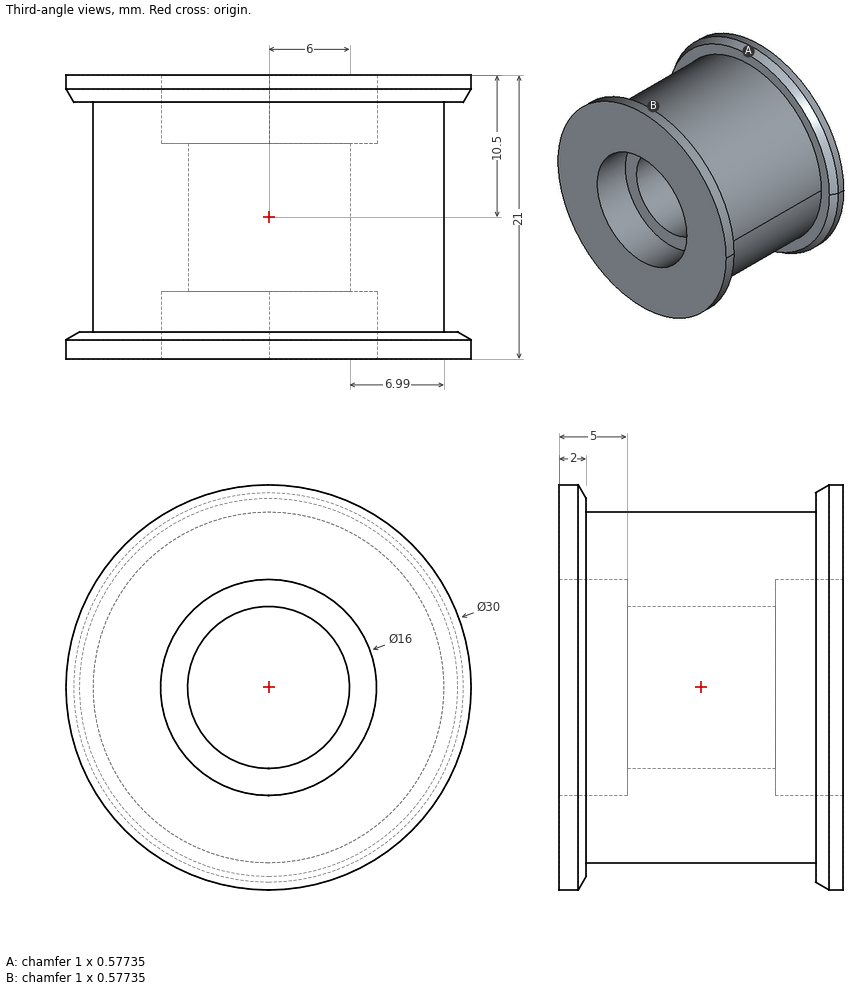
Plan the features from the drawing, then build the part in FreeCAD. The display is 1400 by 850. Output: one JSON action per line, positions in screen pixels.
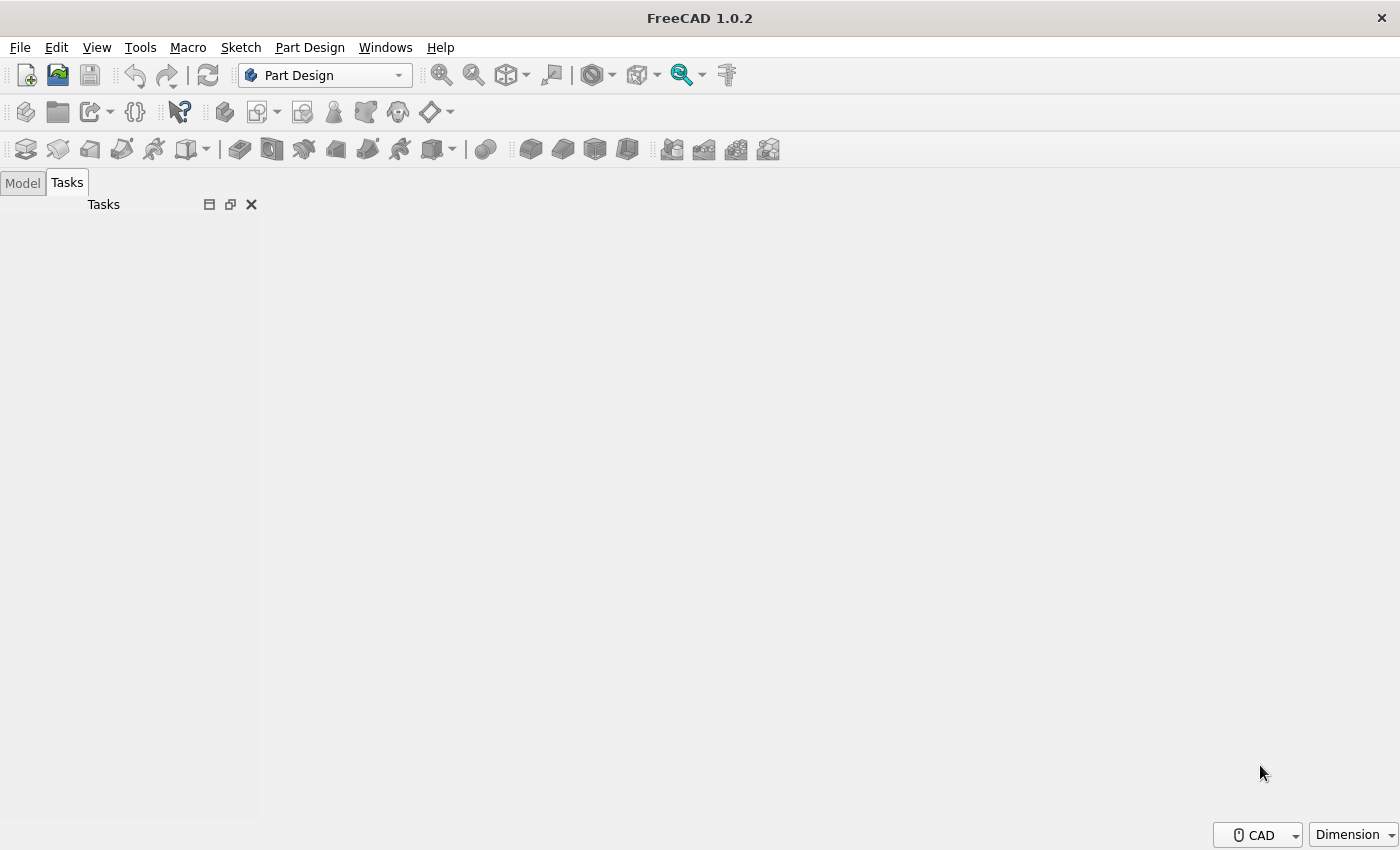
{"action": "left_click", "coordinate": [26, 76]}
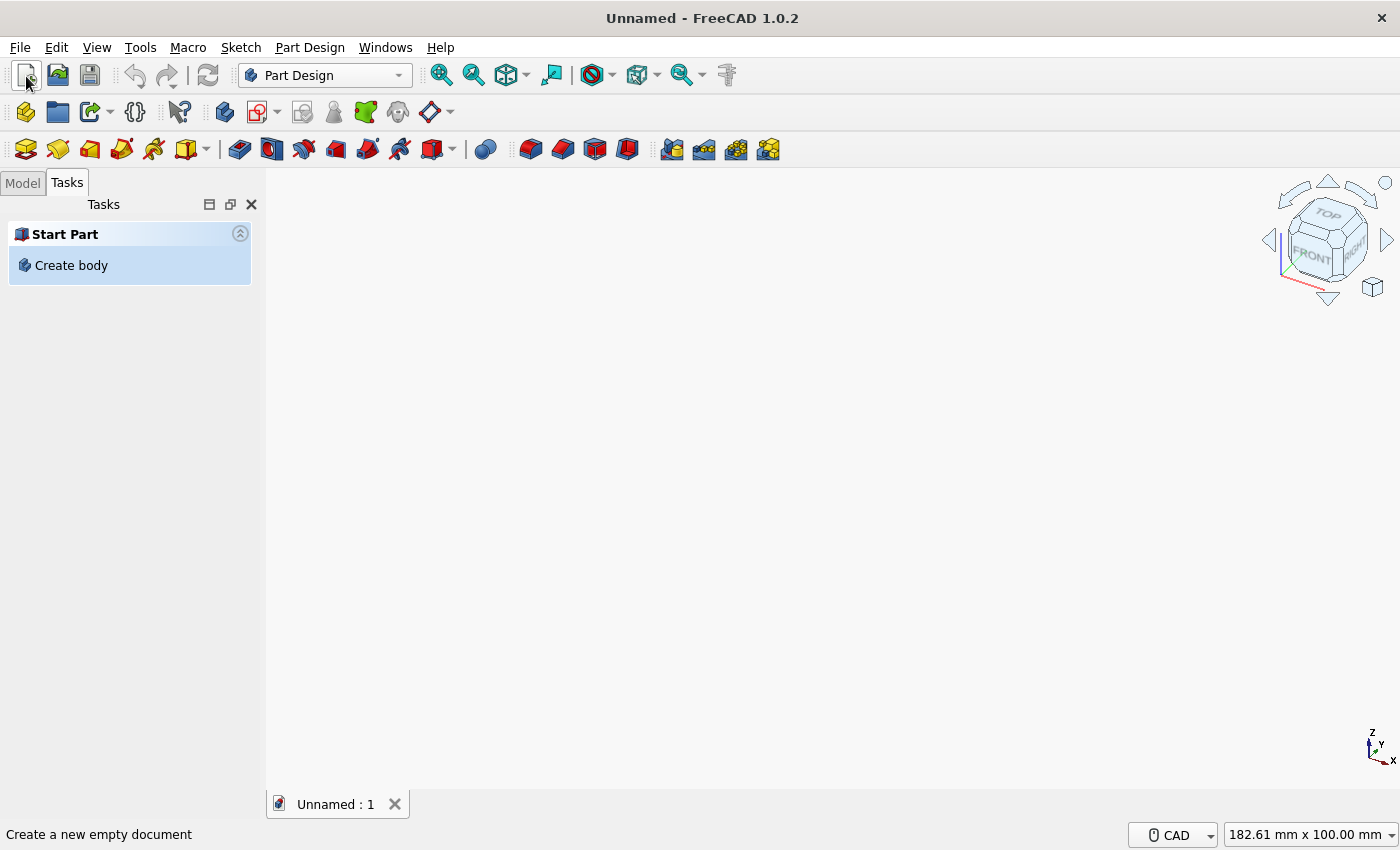
{"action": "left_click", "coordinate": [258, 112]}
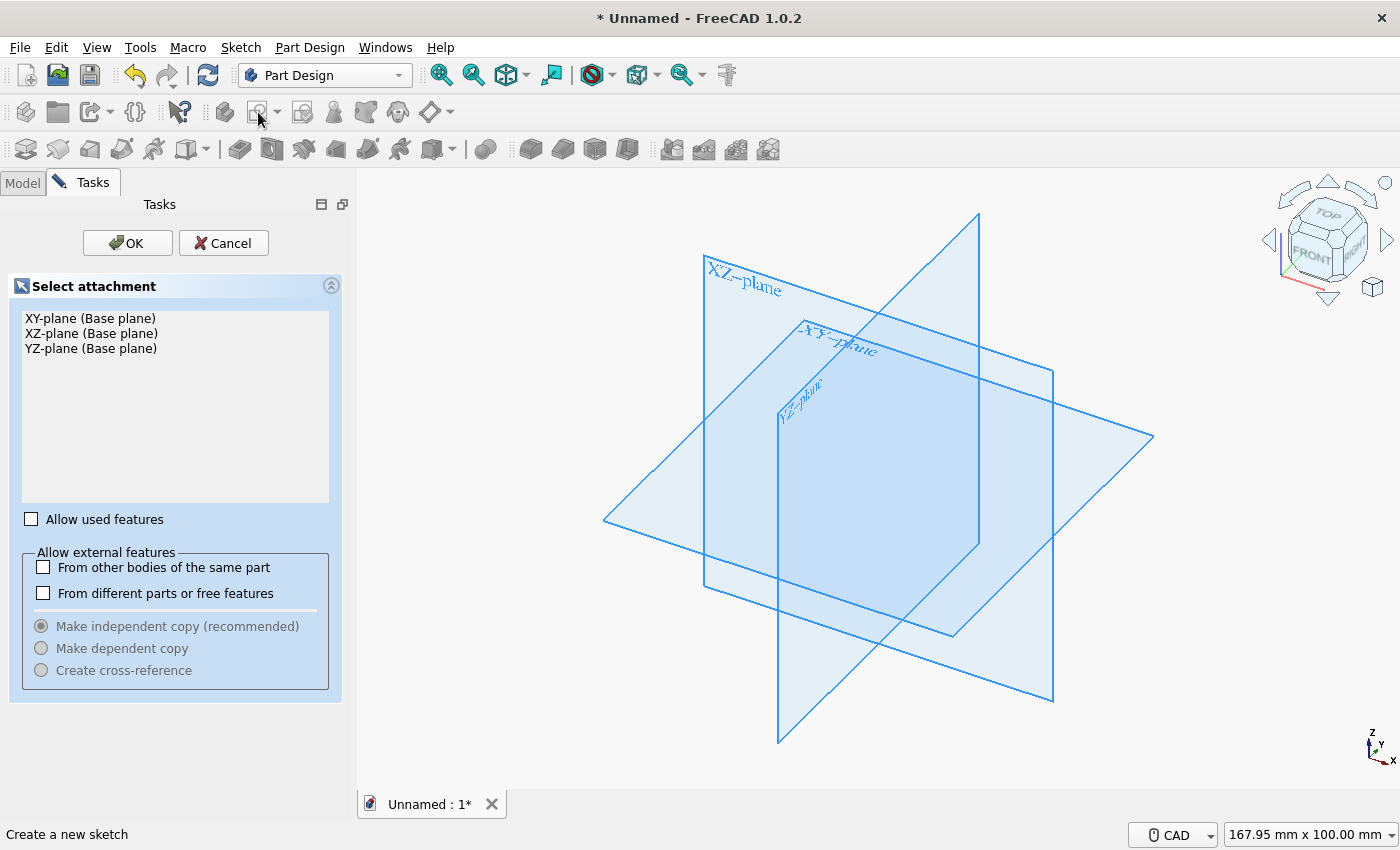
{"action": "left_click", "coordinate": [82, 318]}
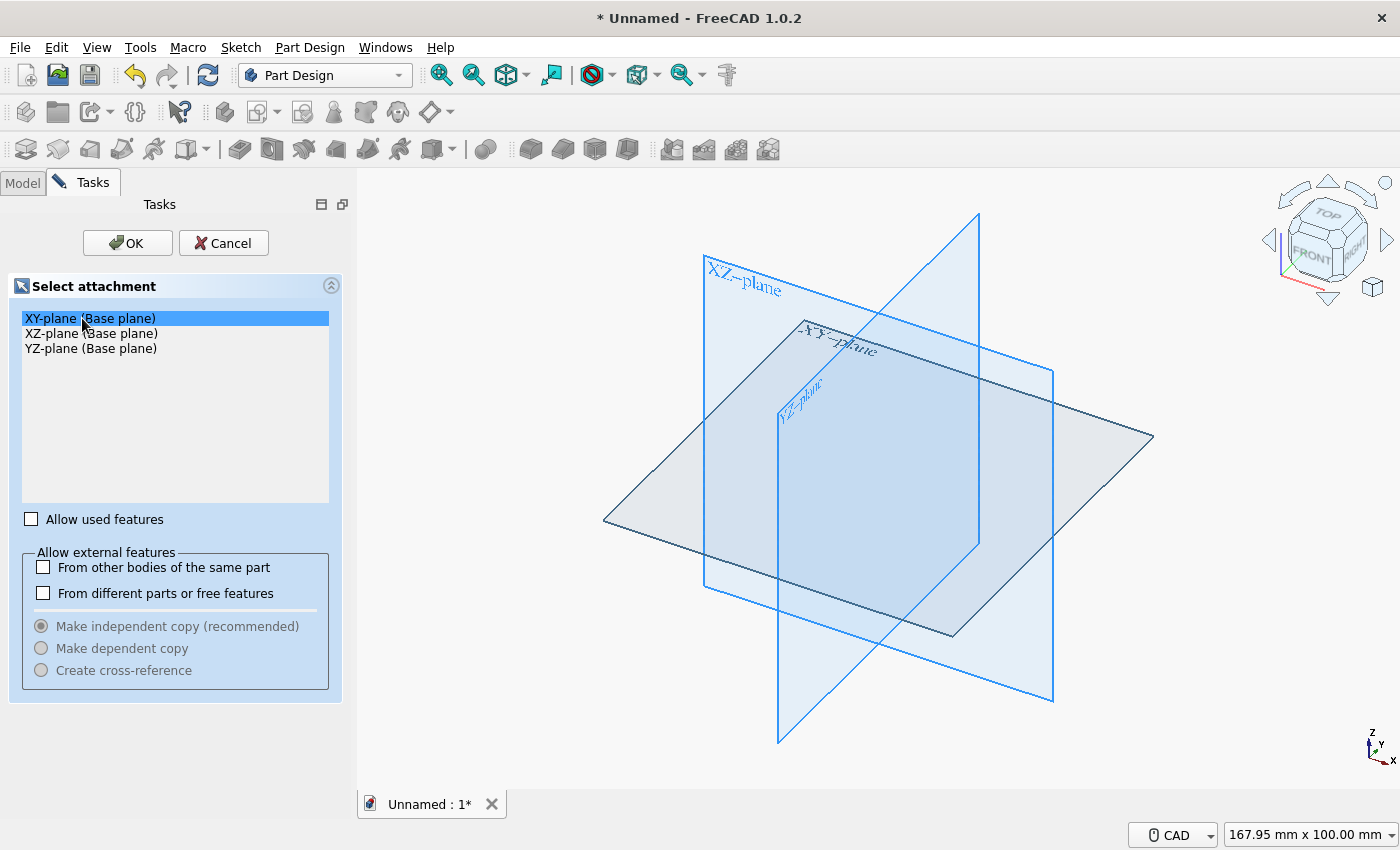
{"action": "left_click", "coordinate": [128, 243]}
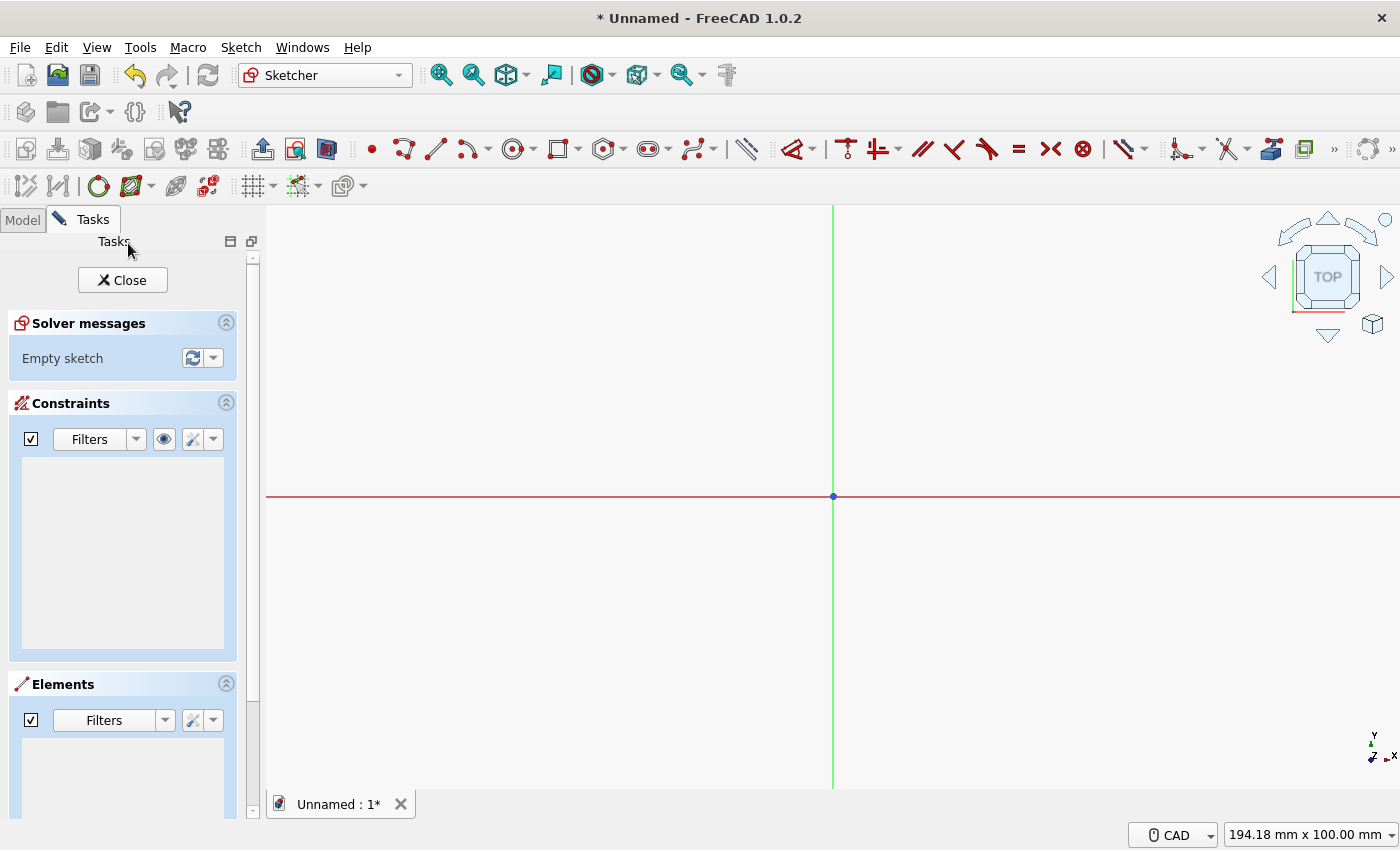
{"action": "scroll", "coordinate": [917, 497], "scroll_direction": "up", "scroll_amount": 6}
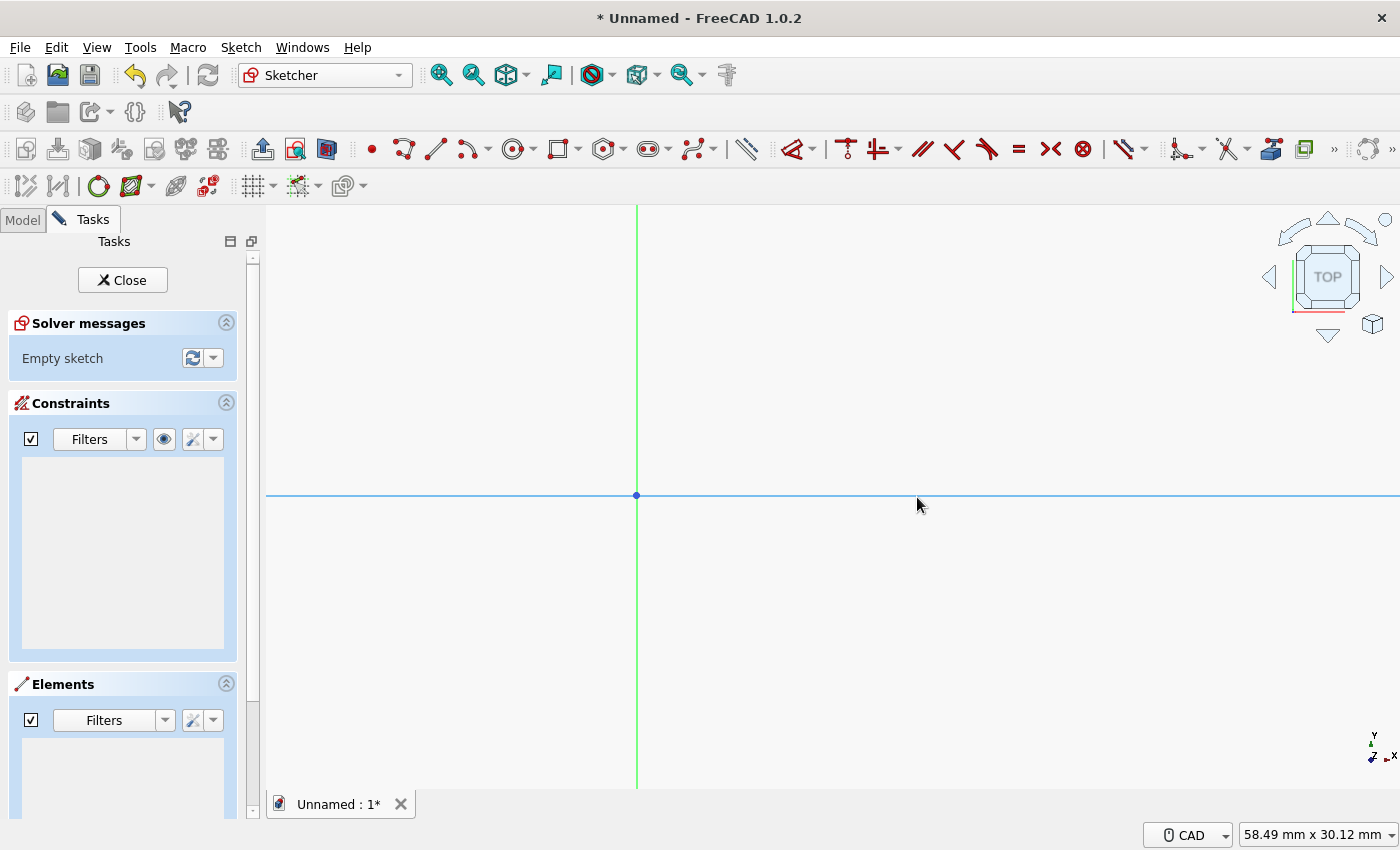
{"action": "left_click", "coordinate": [558, 150]}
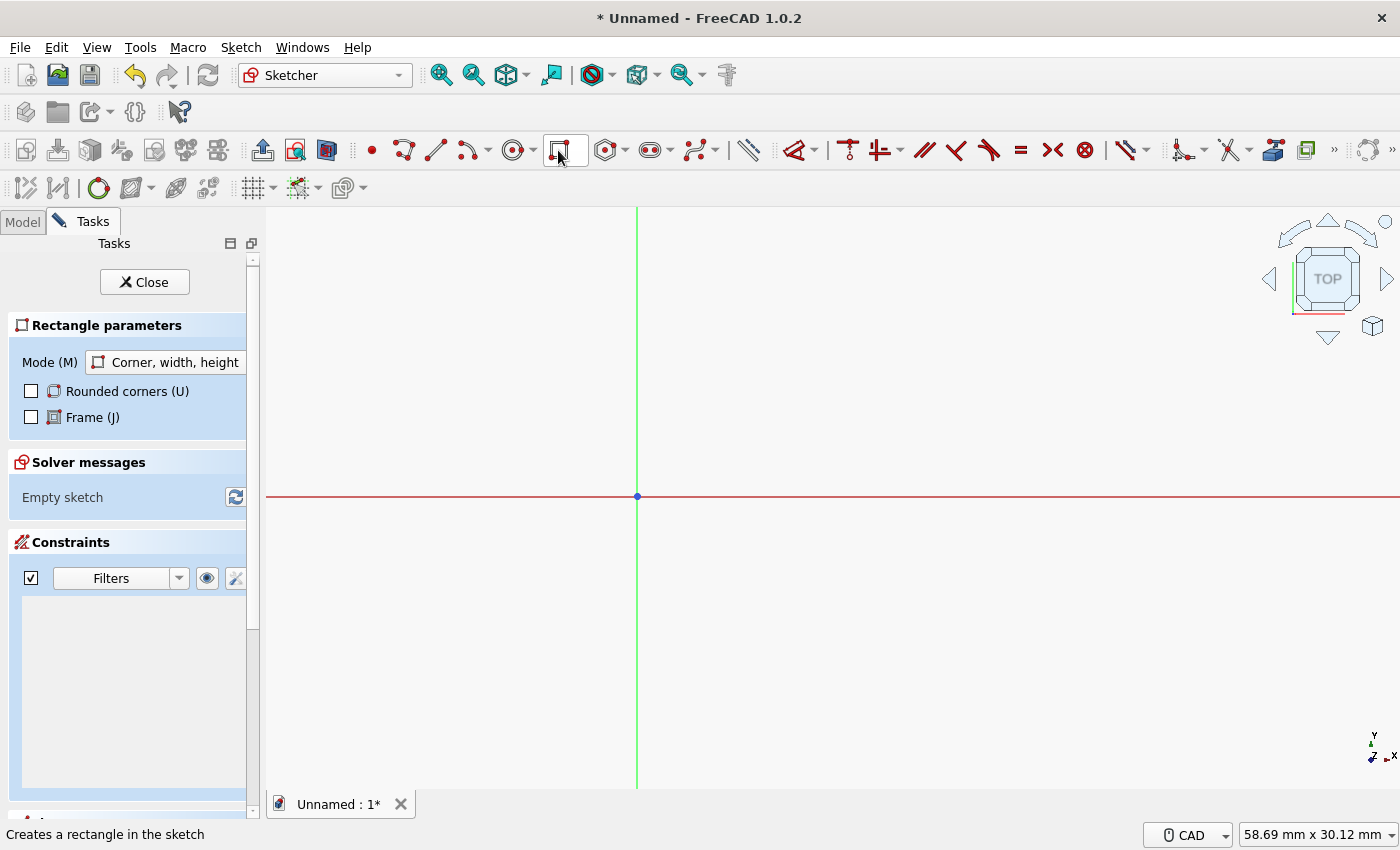
{"action": "left_click", "coordinate": [753, 294]}
{"action": "mouse_move", "coordinate": [888, 700]}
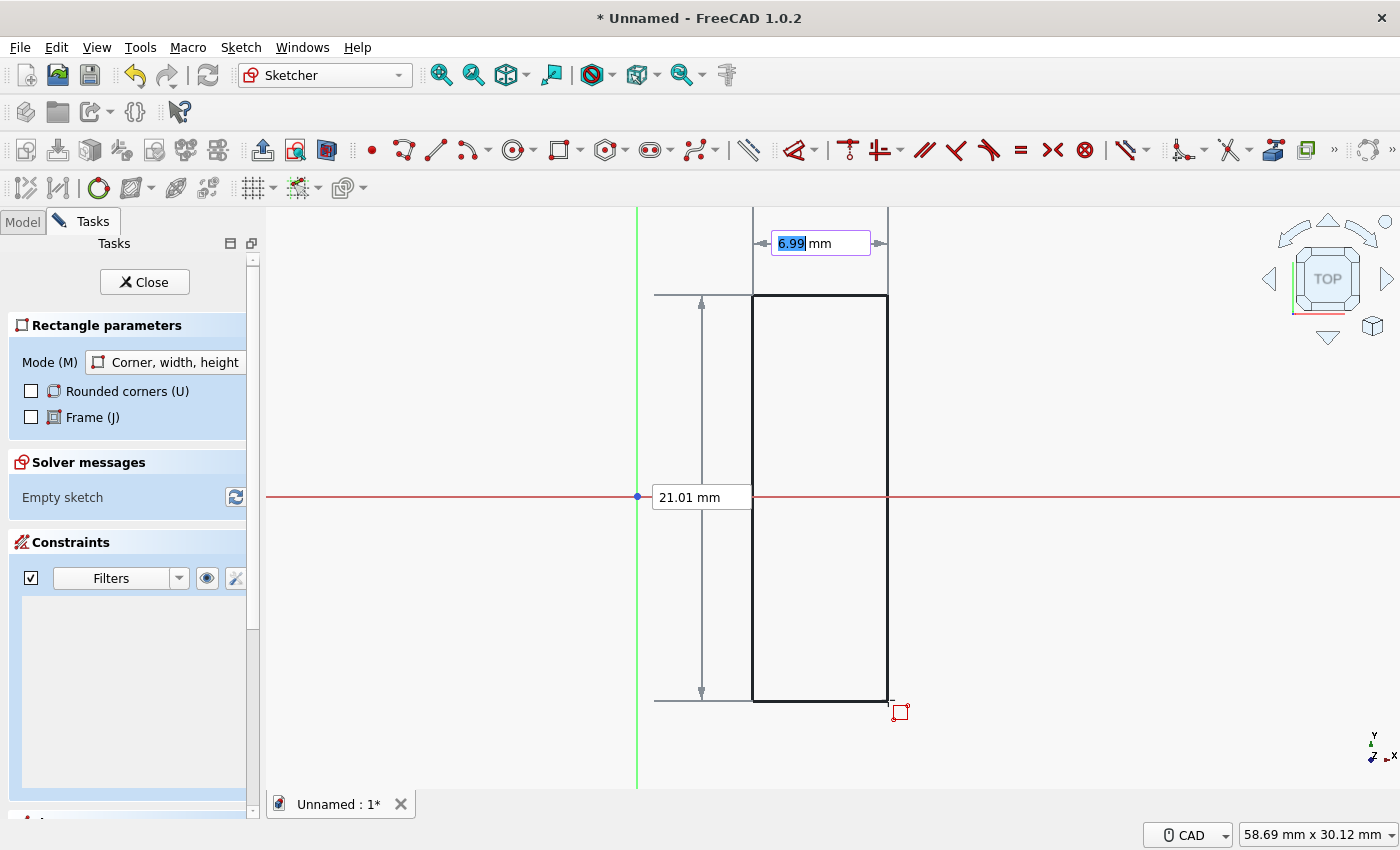
{"action": "type", "text": "6.99"}
{"action": "key", "text": "Tab"}
{"action": "type", "text": "21"}
{"action": "key", "text": "Return"}
{"action": "key", "text": "Escape"}